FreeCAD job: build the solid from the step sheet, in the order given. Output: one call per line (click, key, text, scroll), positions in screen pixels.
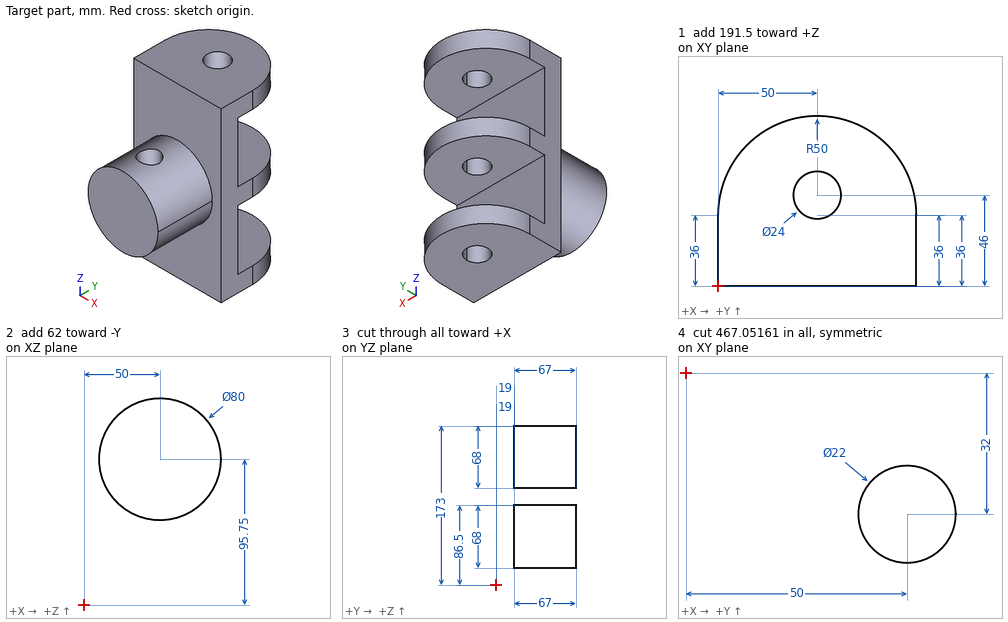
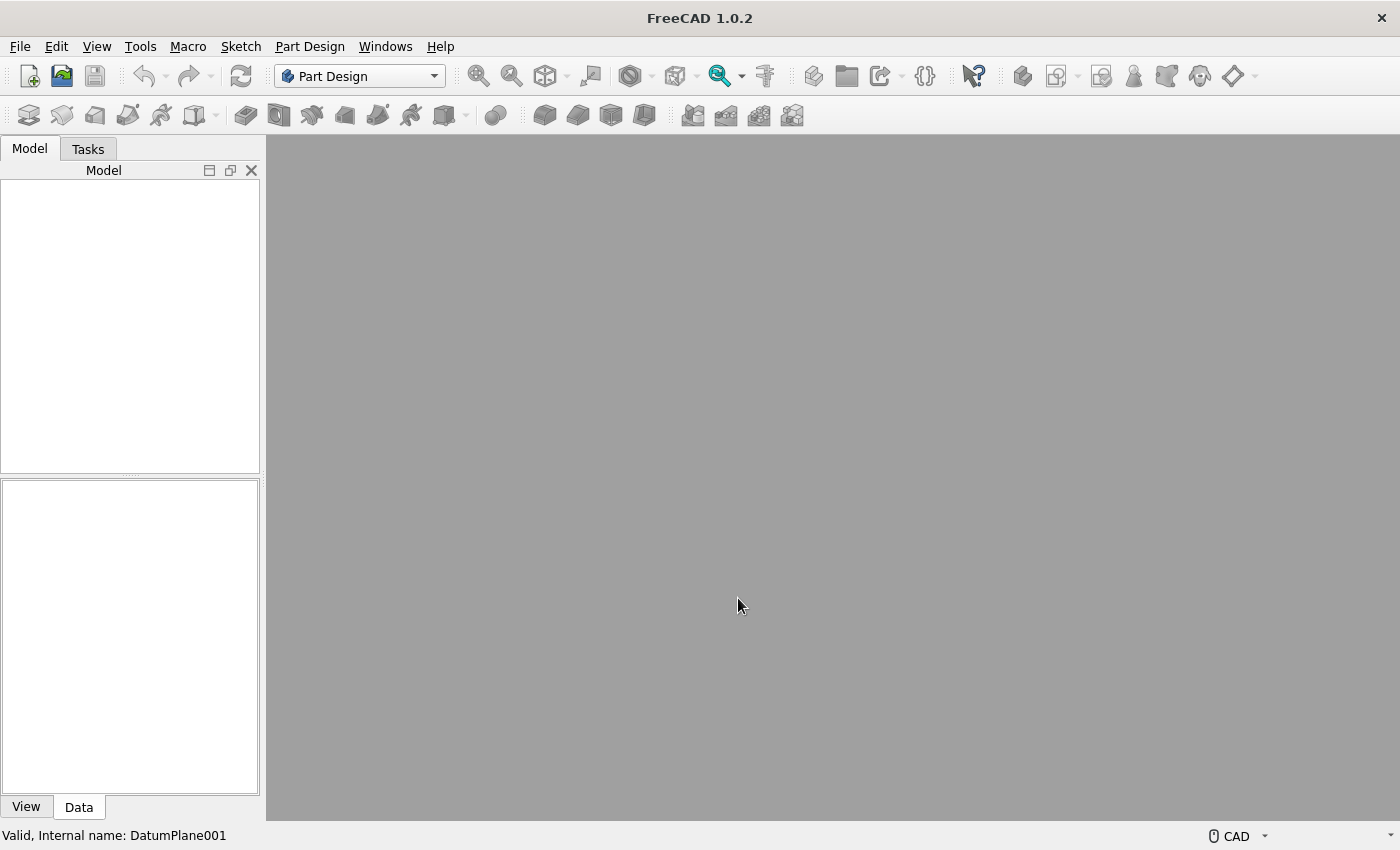
click(29, 76)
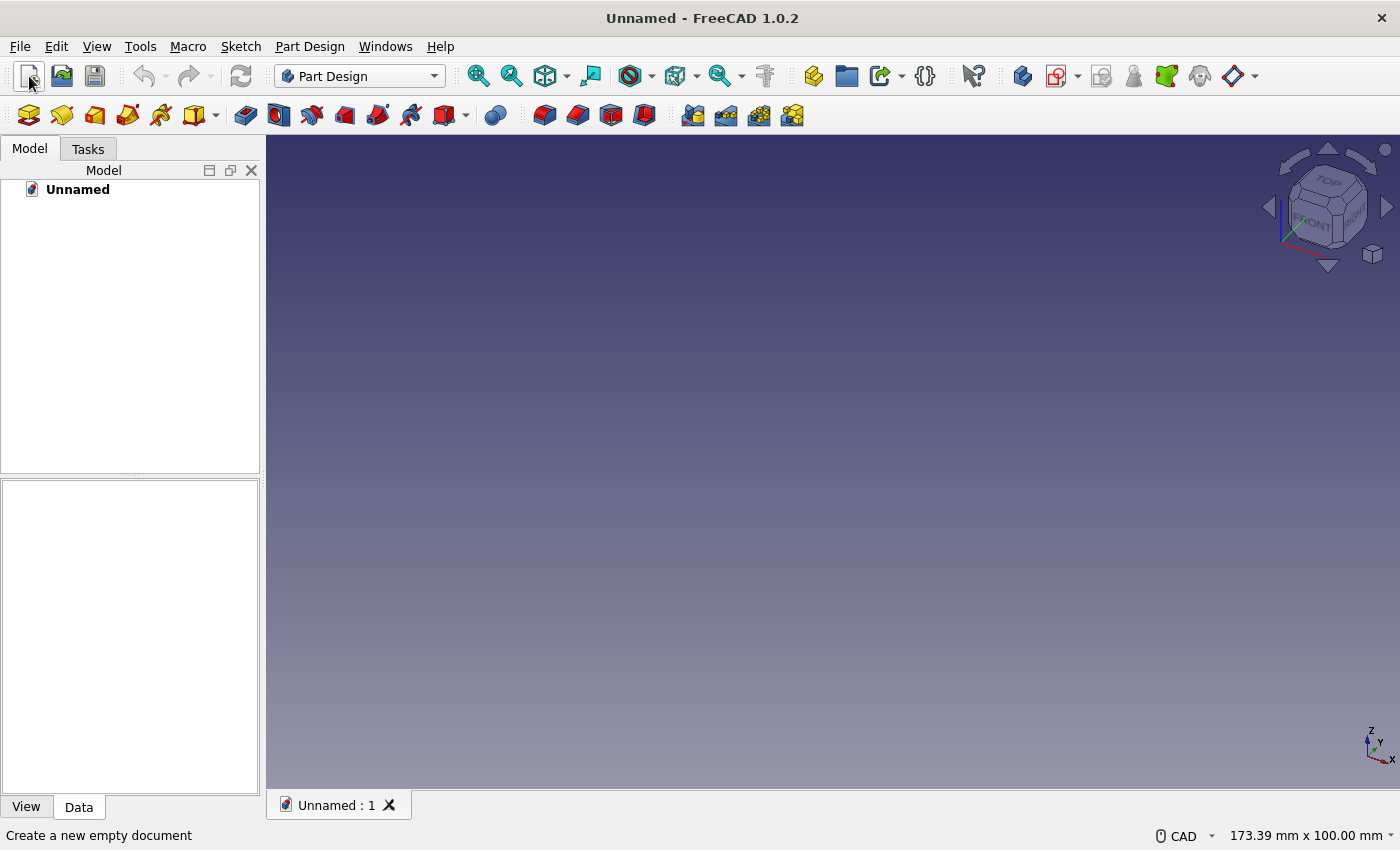
click(1056, 76)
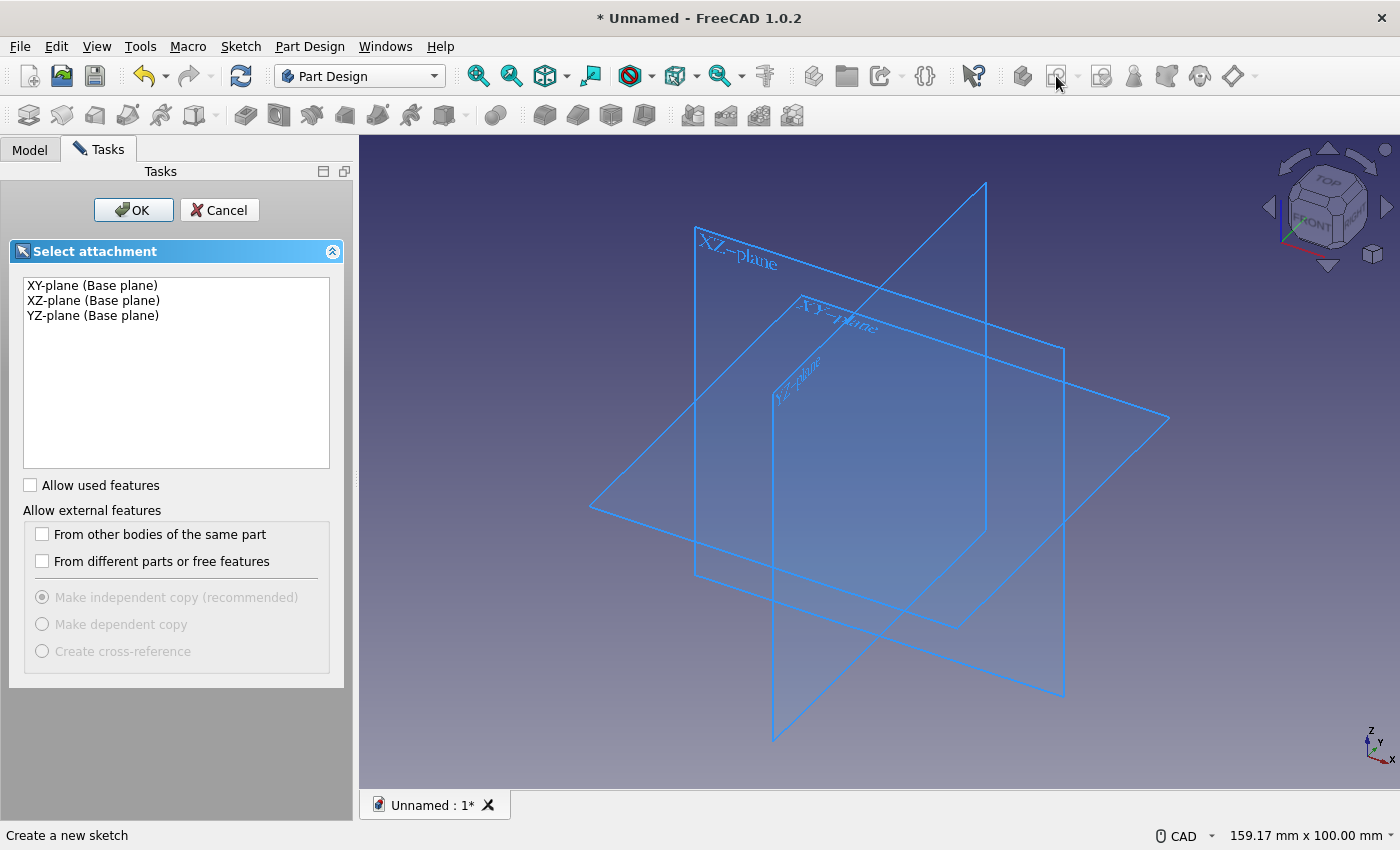
click(84, 286)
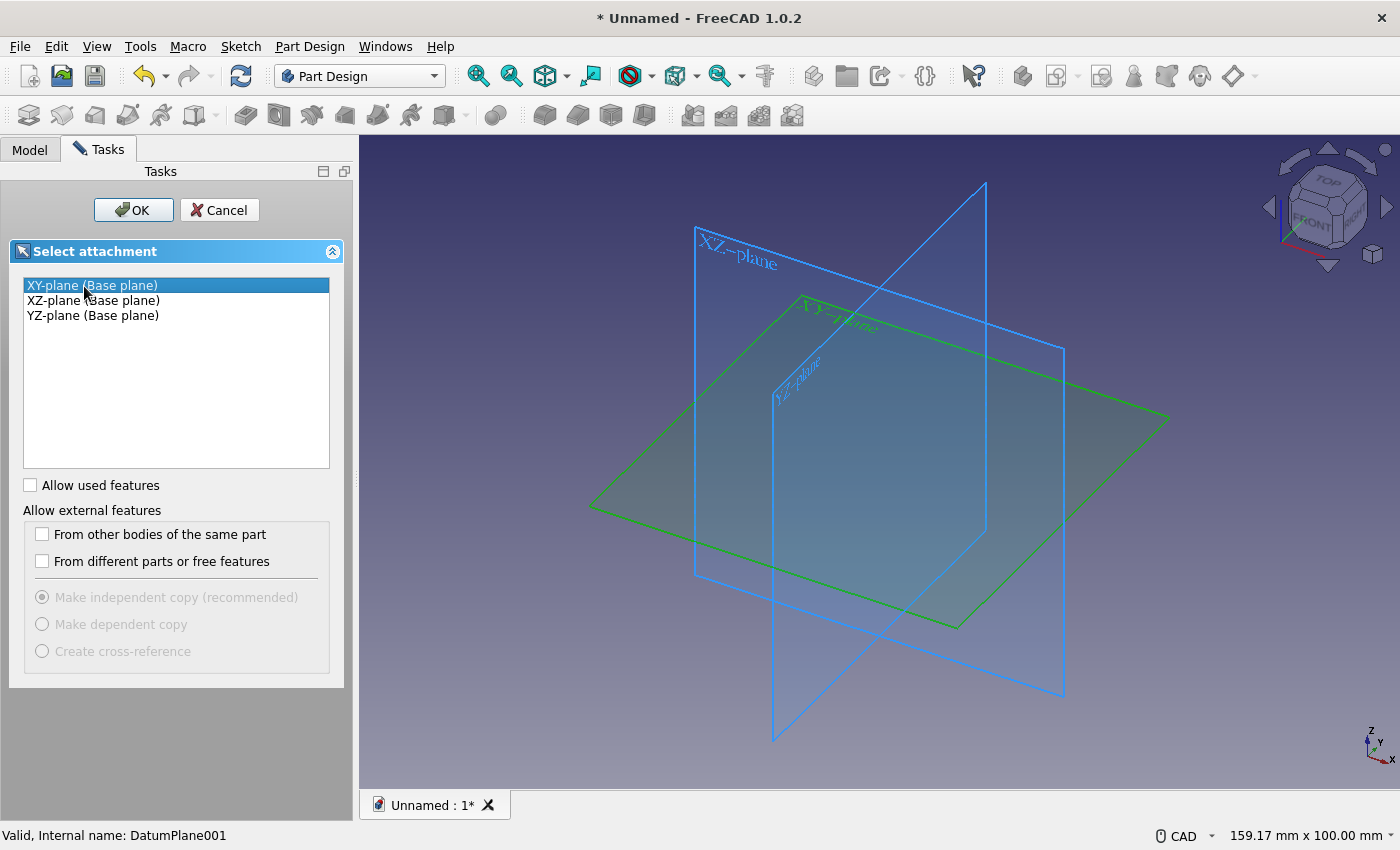
click(134, 210)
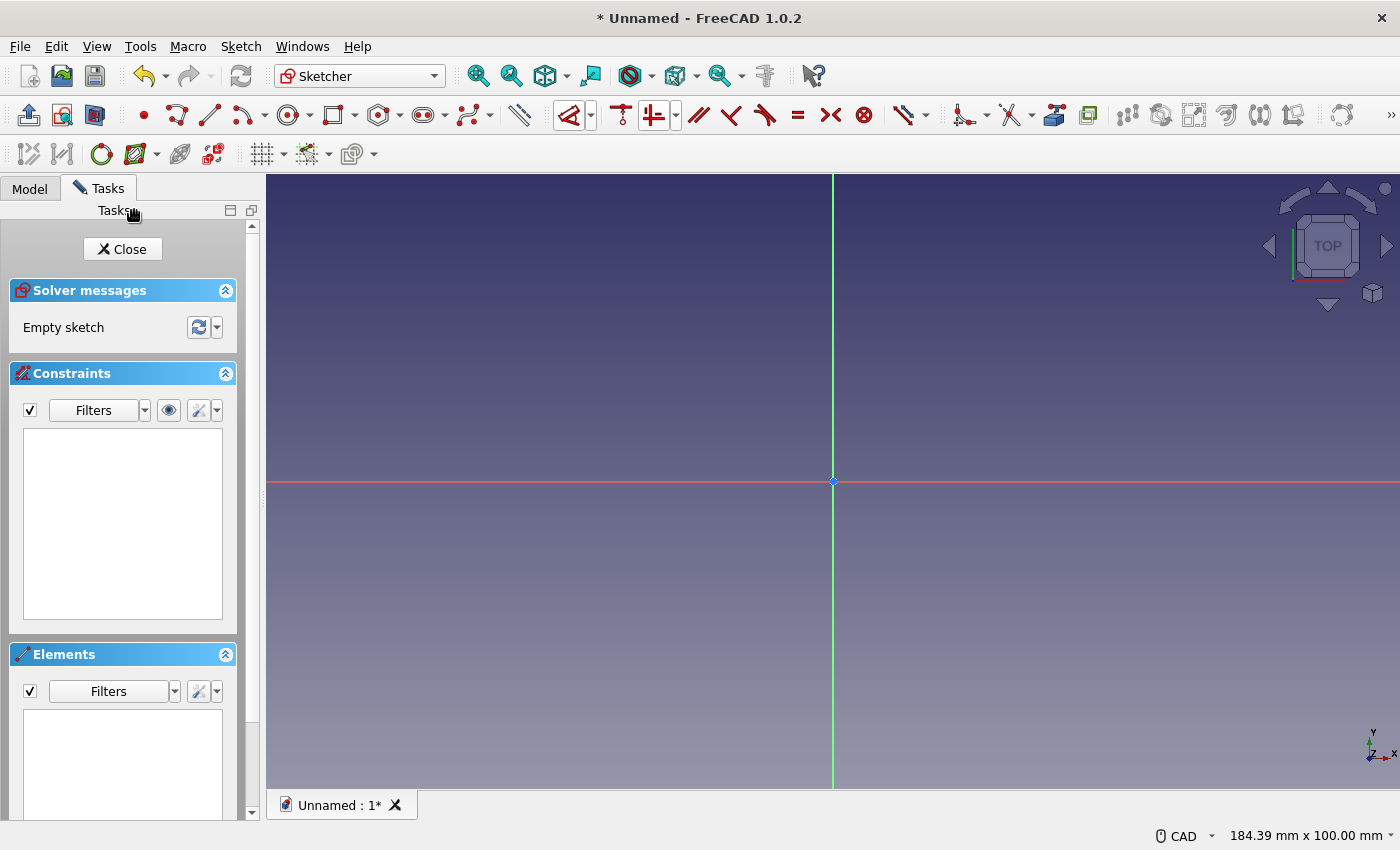
scroll(307, 761, down, 3)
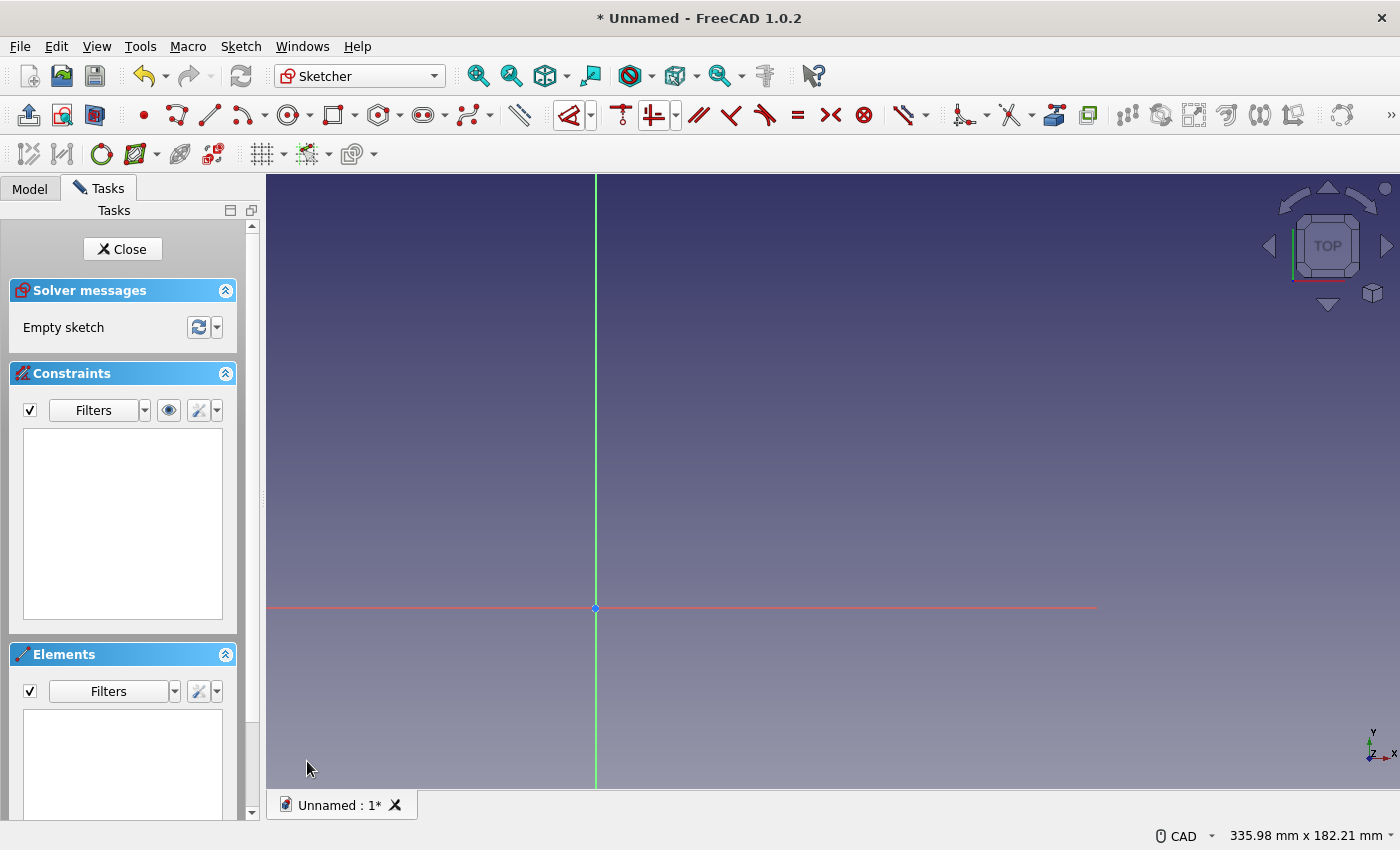
scroll(764, 425, up, 2)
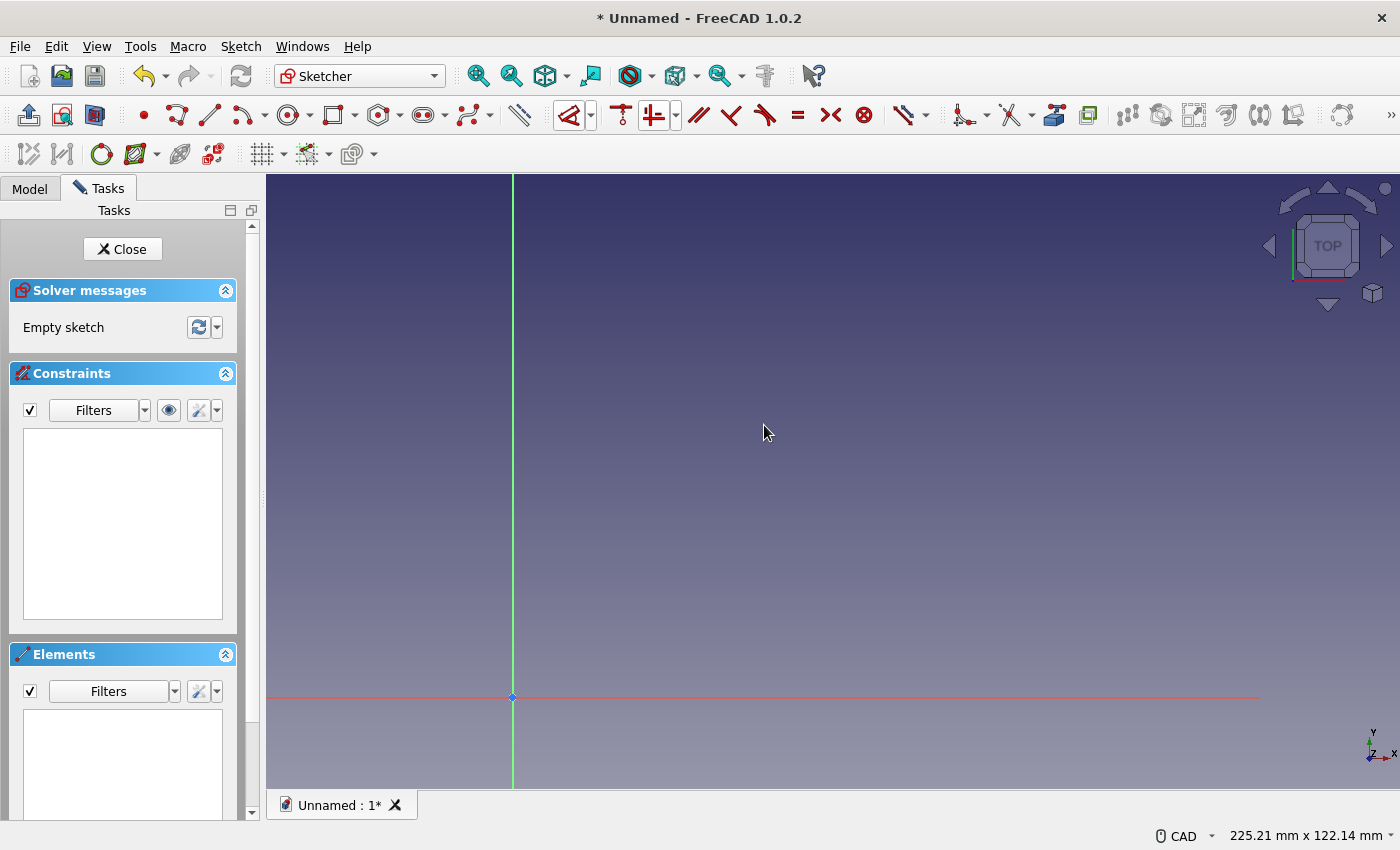
click(177, 116)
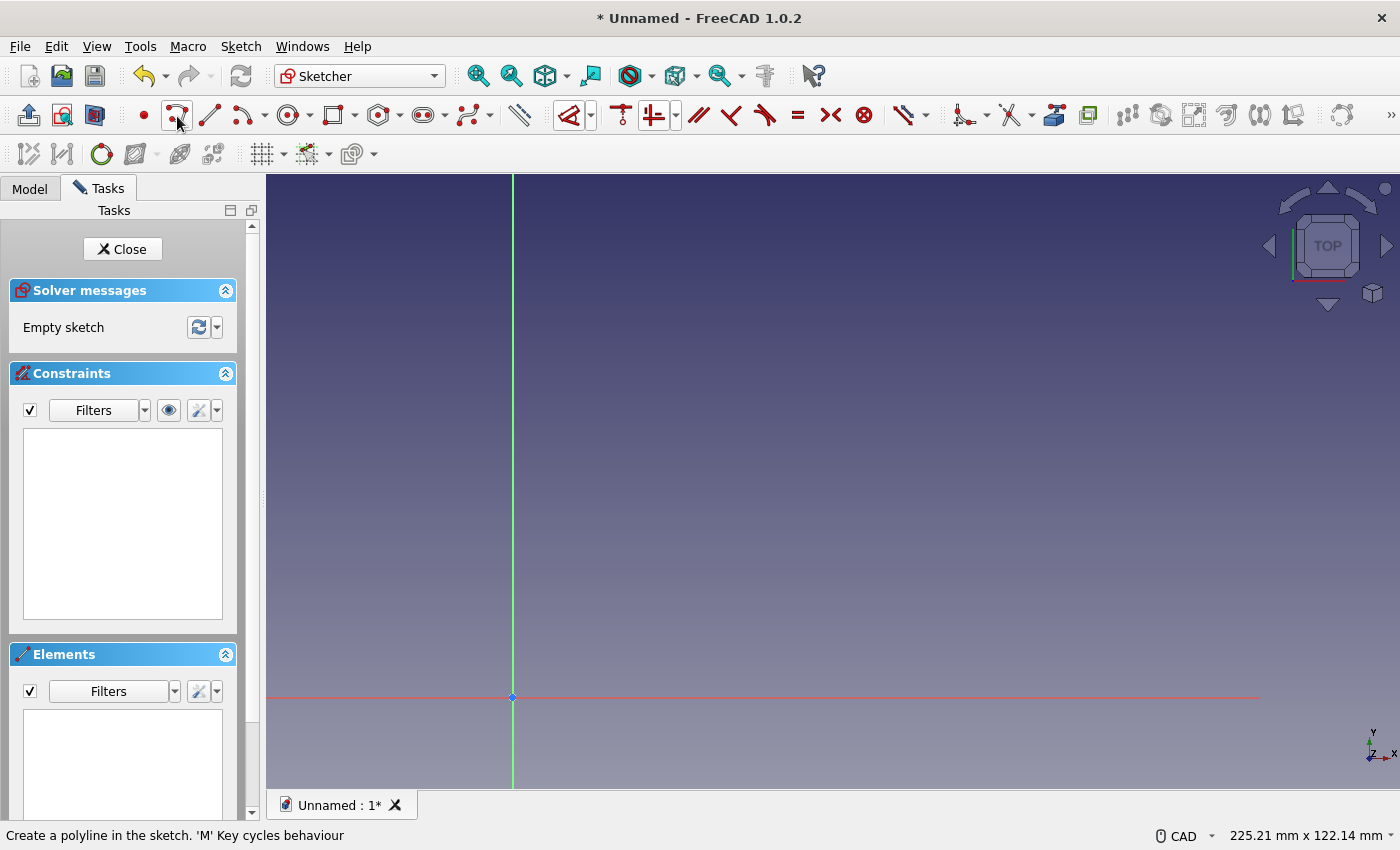
click(513, 517)
click(513, 698)
click(1016, 689)
click(1016, 517)
right_click(1016, 517)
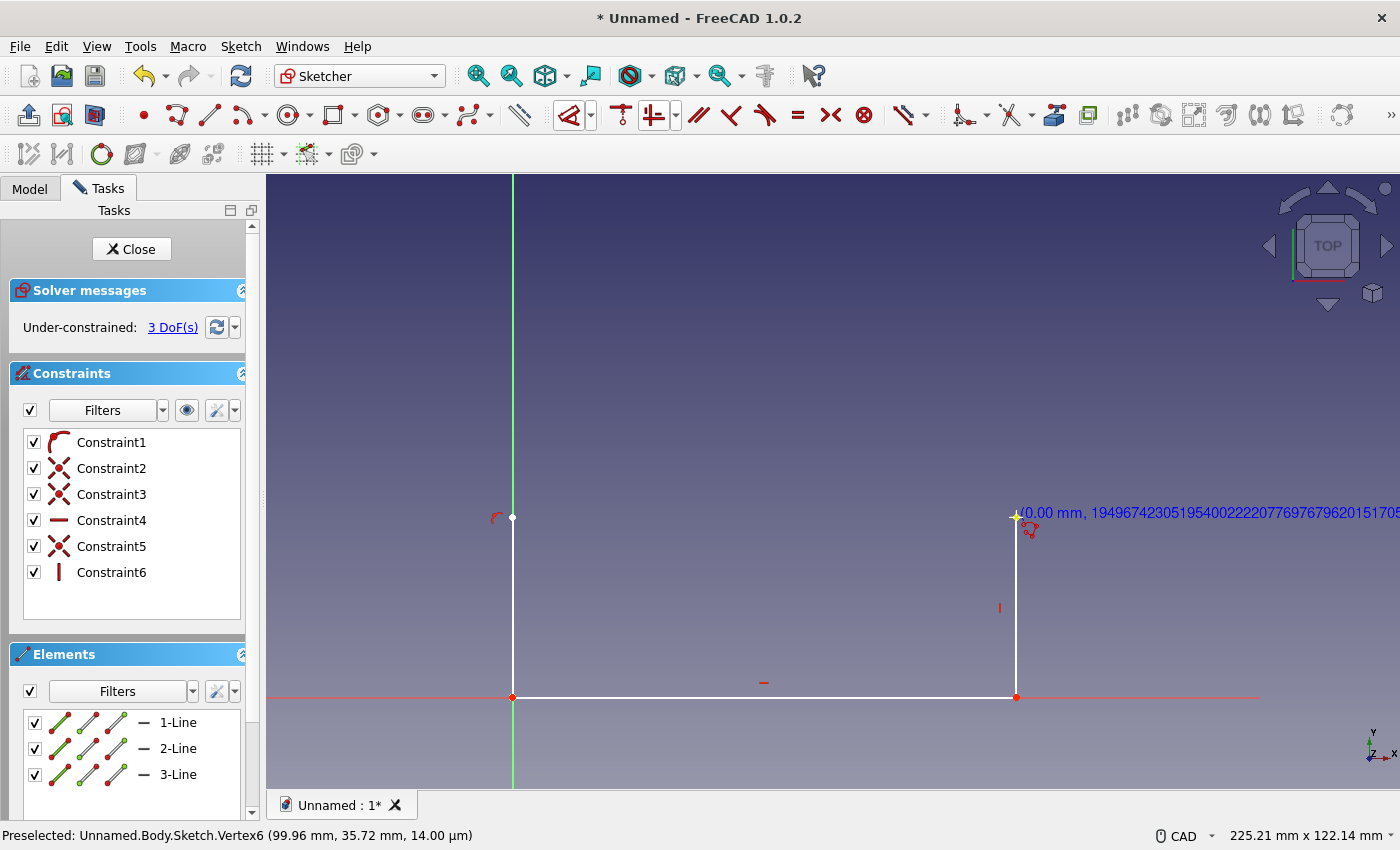
click(264, 116)